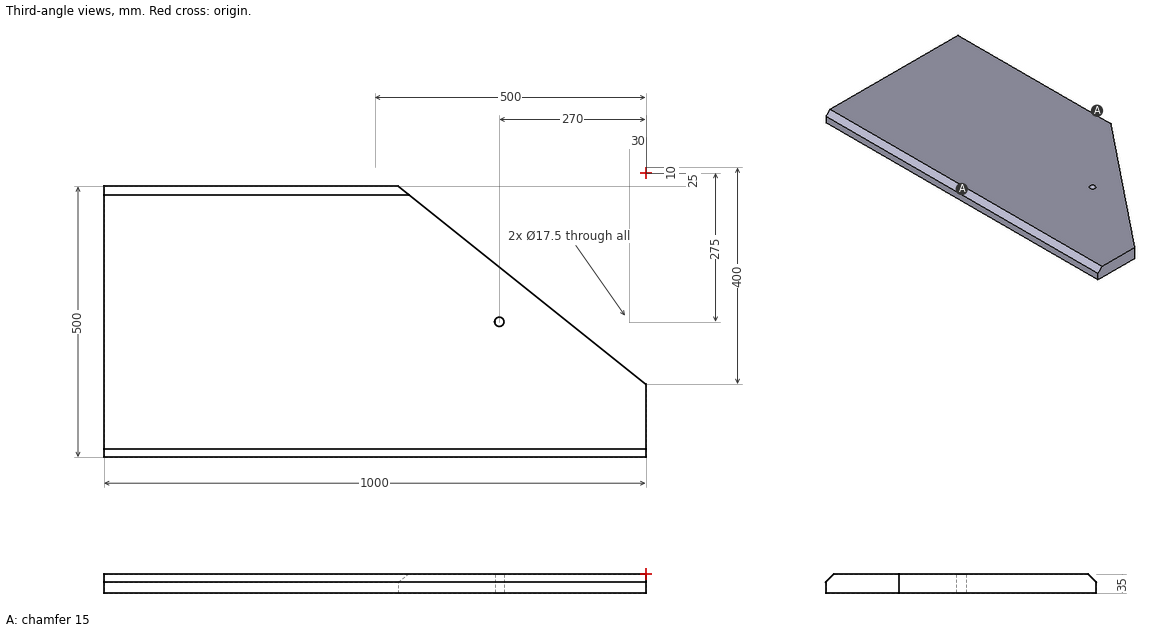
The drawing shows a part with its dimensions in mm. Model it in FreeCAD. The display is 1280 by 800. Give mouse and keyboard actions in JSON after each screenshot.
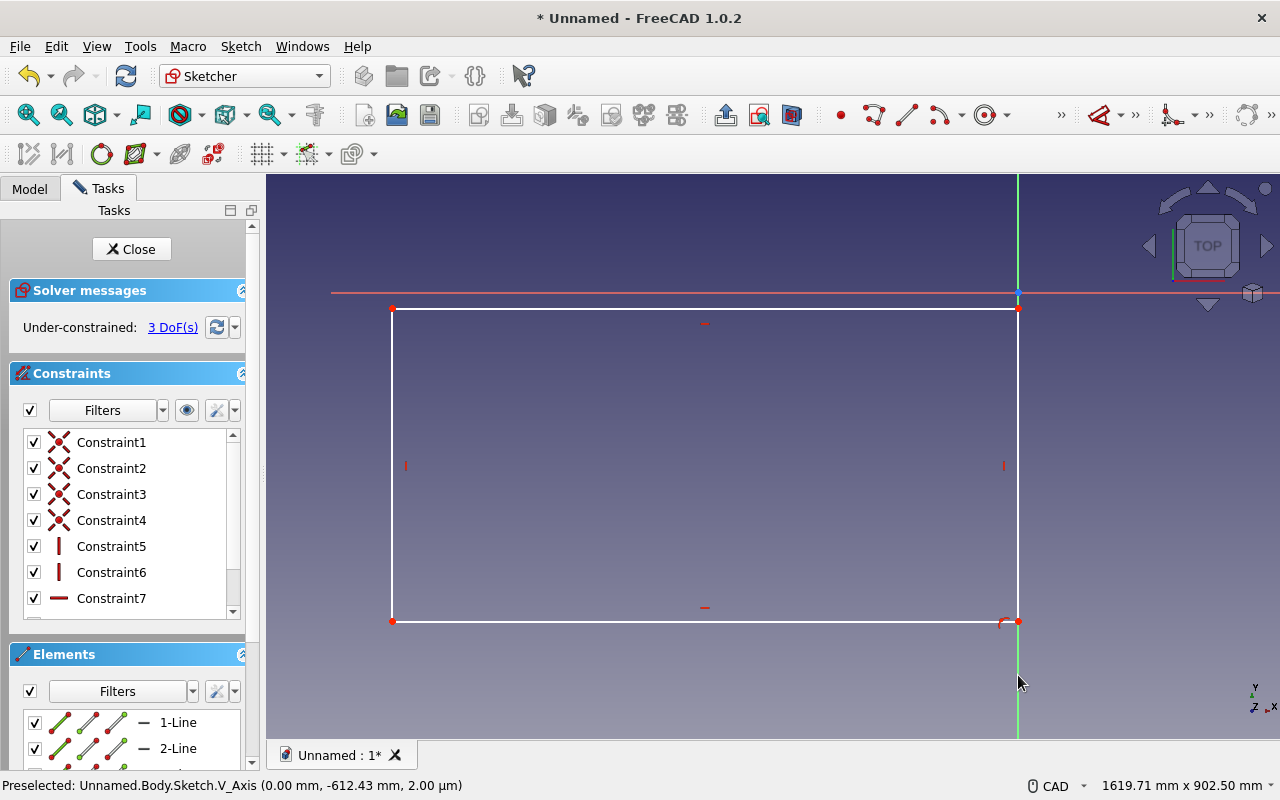
{"action": "left_click", "coordinate": [1098, 116]}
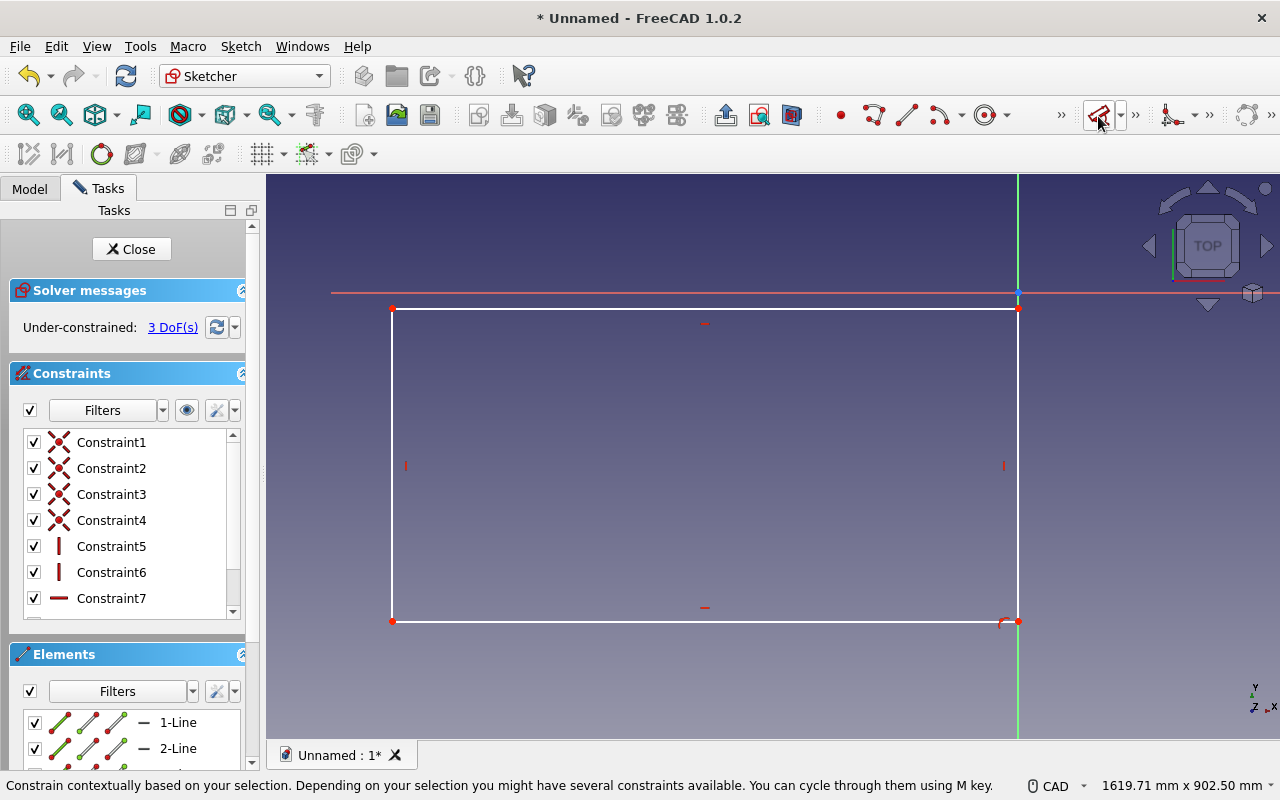
{"action": "left_click", "coordinate": [392, 403]}
{"action": "left_click", "coordinate": [358, 465]}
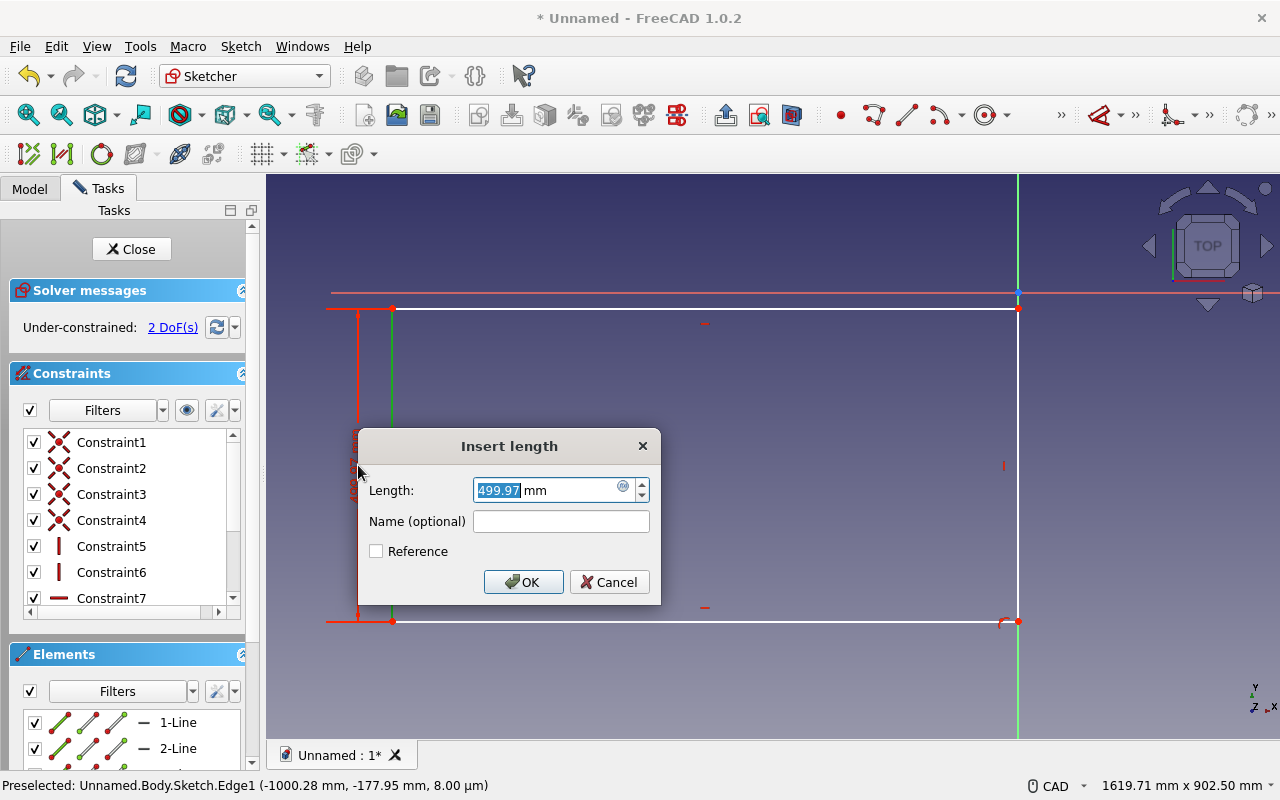
{"action": "type", "text": "500"}
{"action": "key", "text": "Return"}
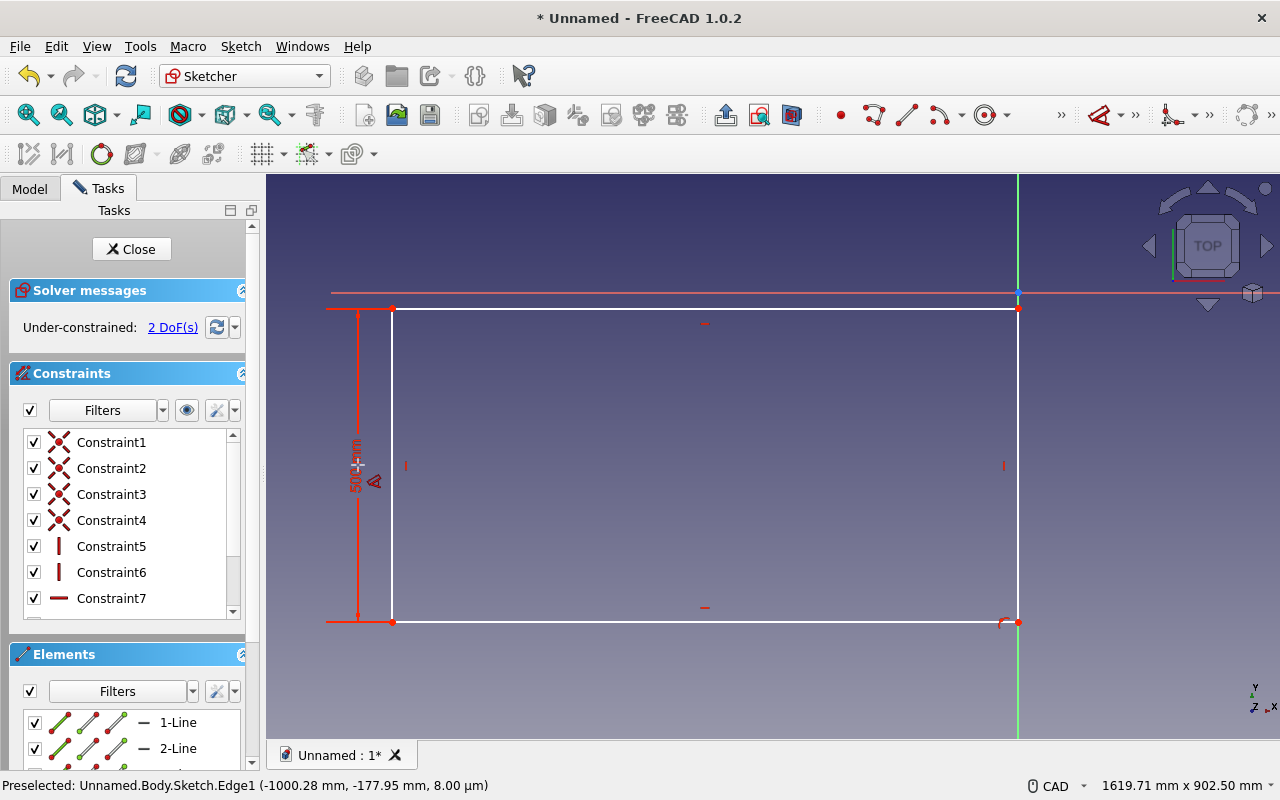
{"action": "scroll", "coordinate": [392, 309], "scroll_direction": "up", "scroll_amount": 5}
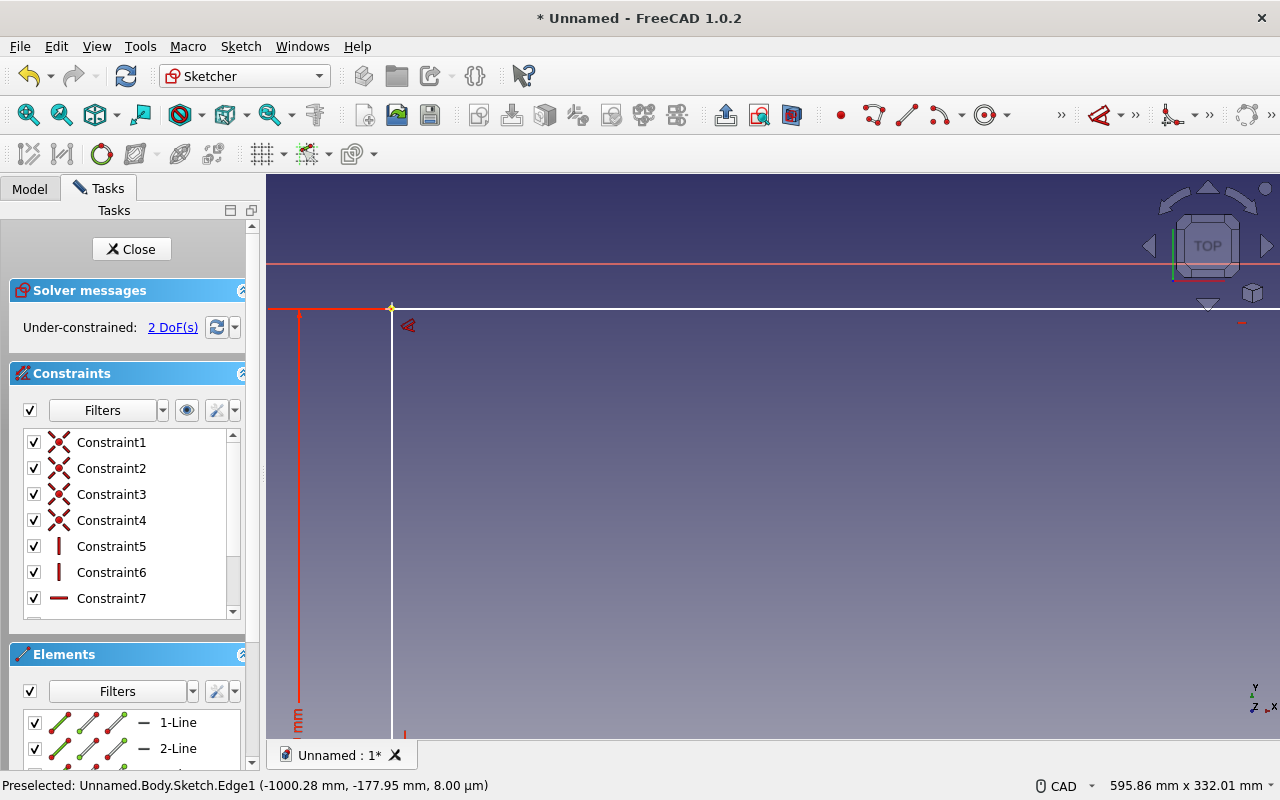
{"action": "left_click", "coordinate": [392, 309]}
{"action": "left_click", "coordinate": [358, 286]}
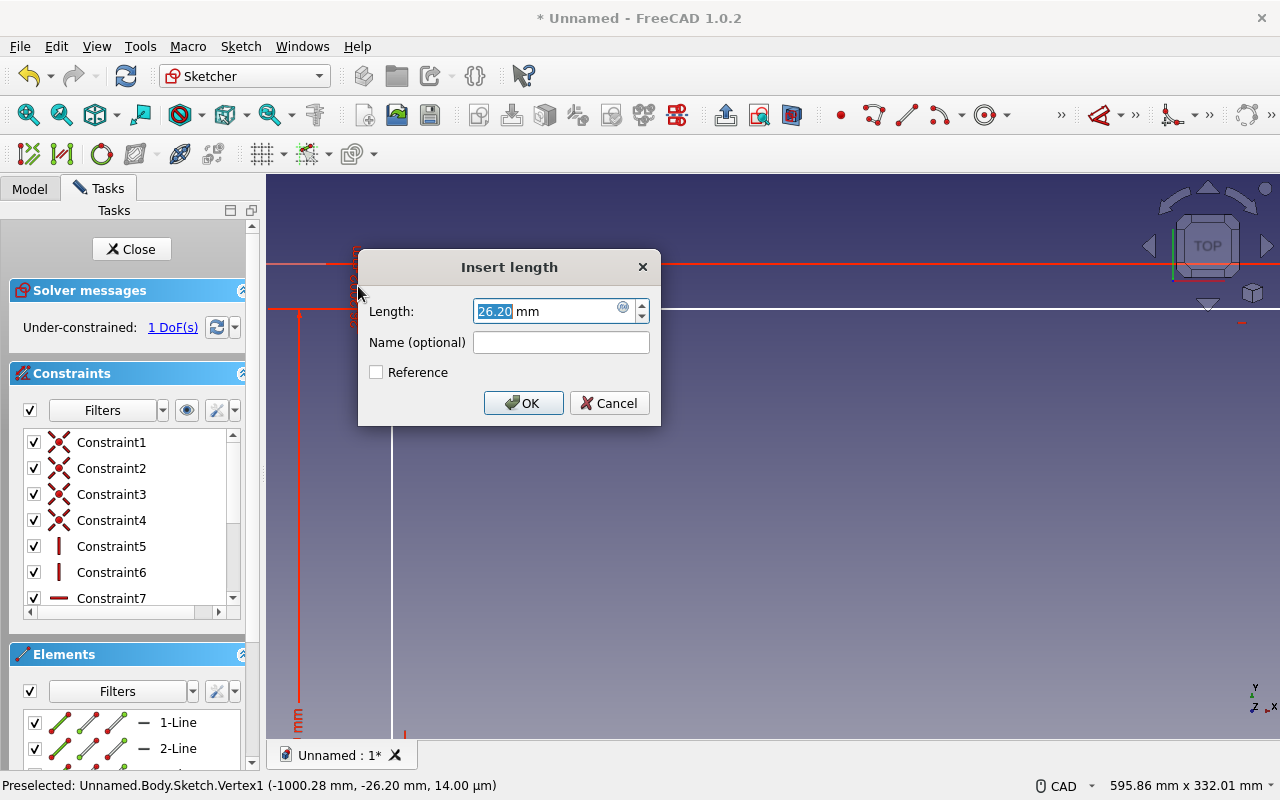
{"action": "type", "text": "25"}
{"action": "key", "text": "Return"}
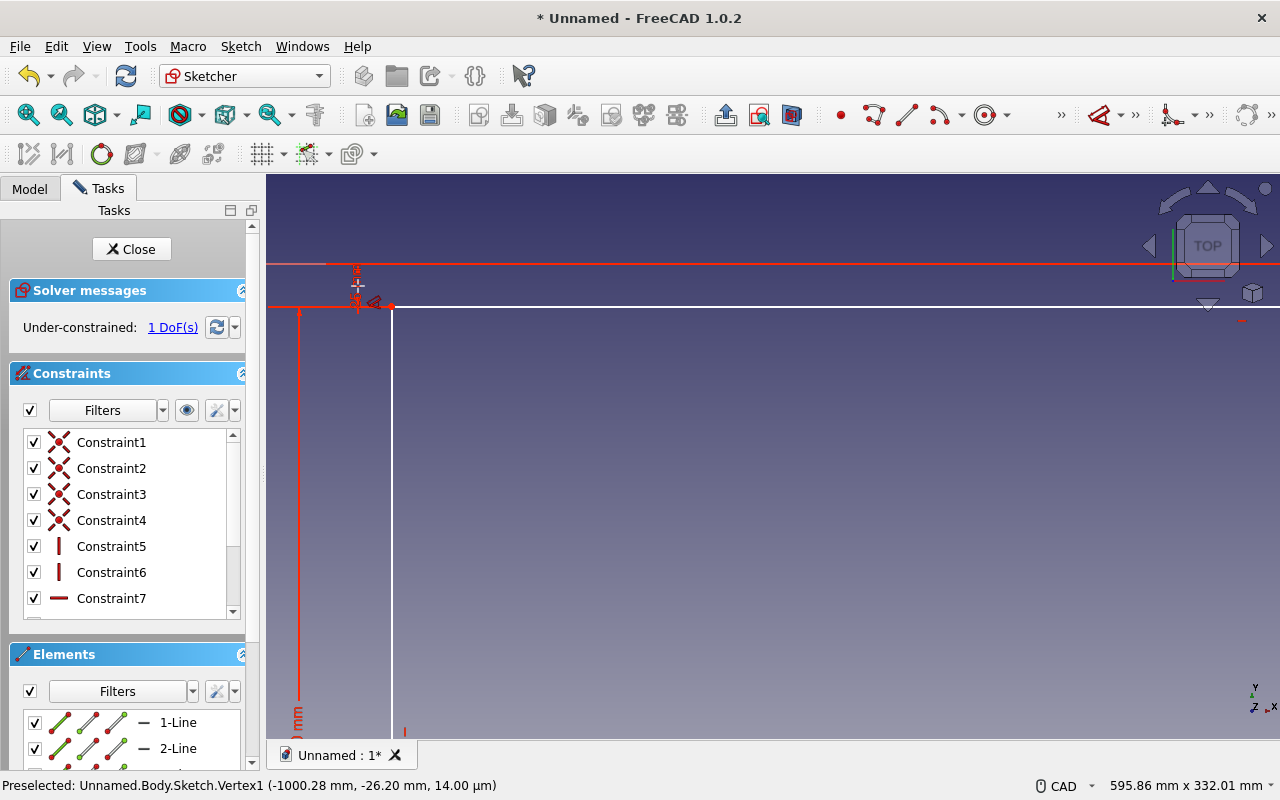
{"action": "scroll", "coordinate": [391, 309], "scroll_direction": "down", "scroll_amount": 5}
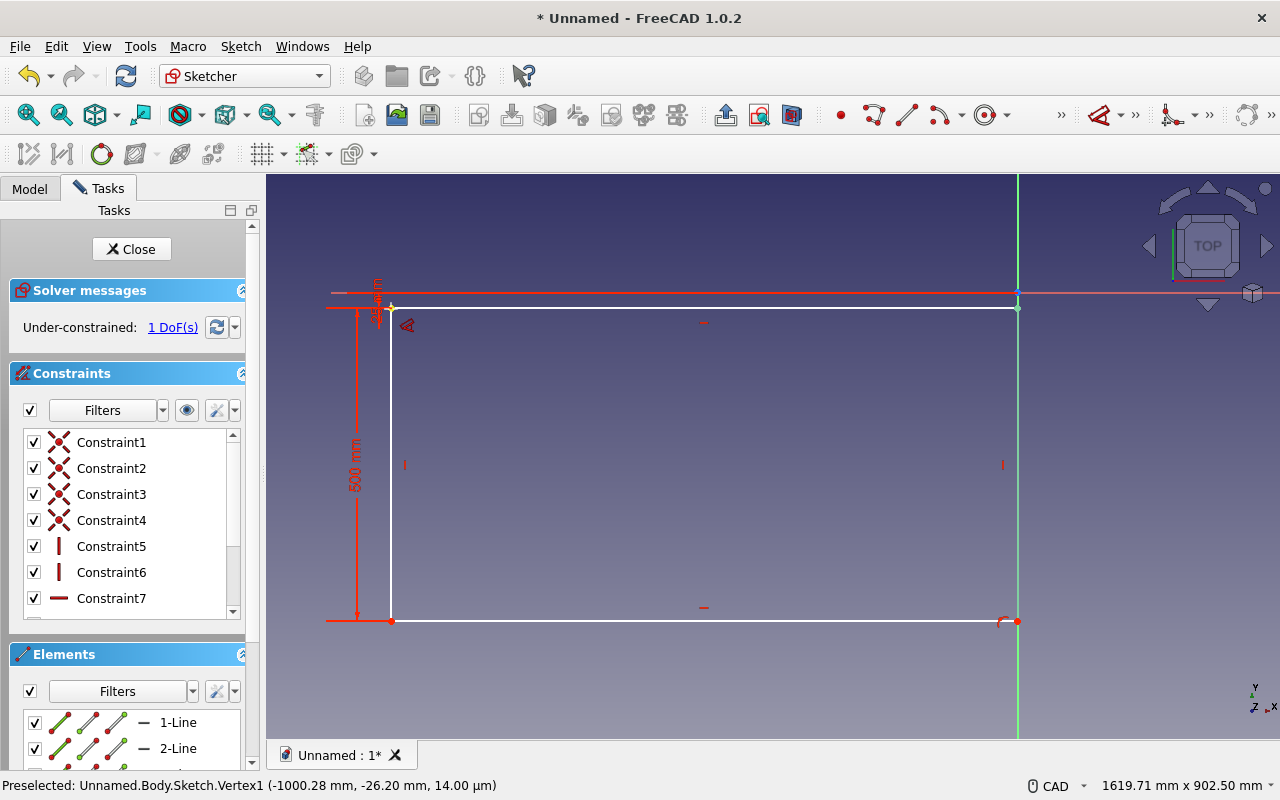
{"action": "left_click", "coordinate": [579, 621]}
{"action": "left_click", "coordinate": [704, 655]}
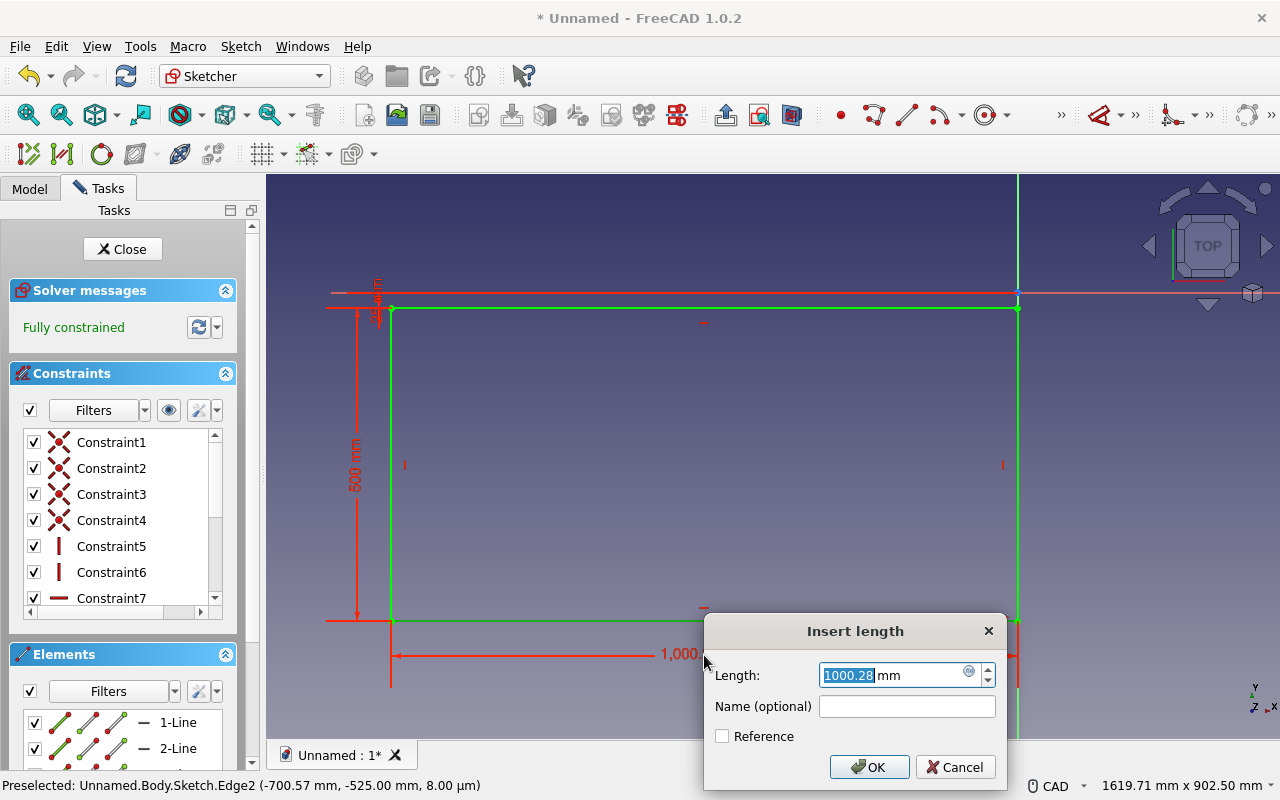
{"action": "type", "text": "1000"}
{"action": "key", "text": "Return"}
{"action": "key", "text": "Escape"}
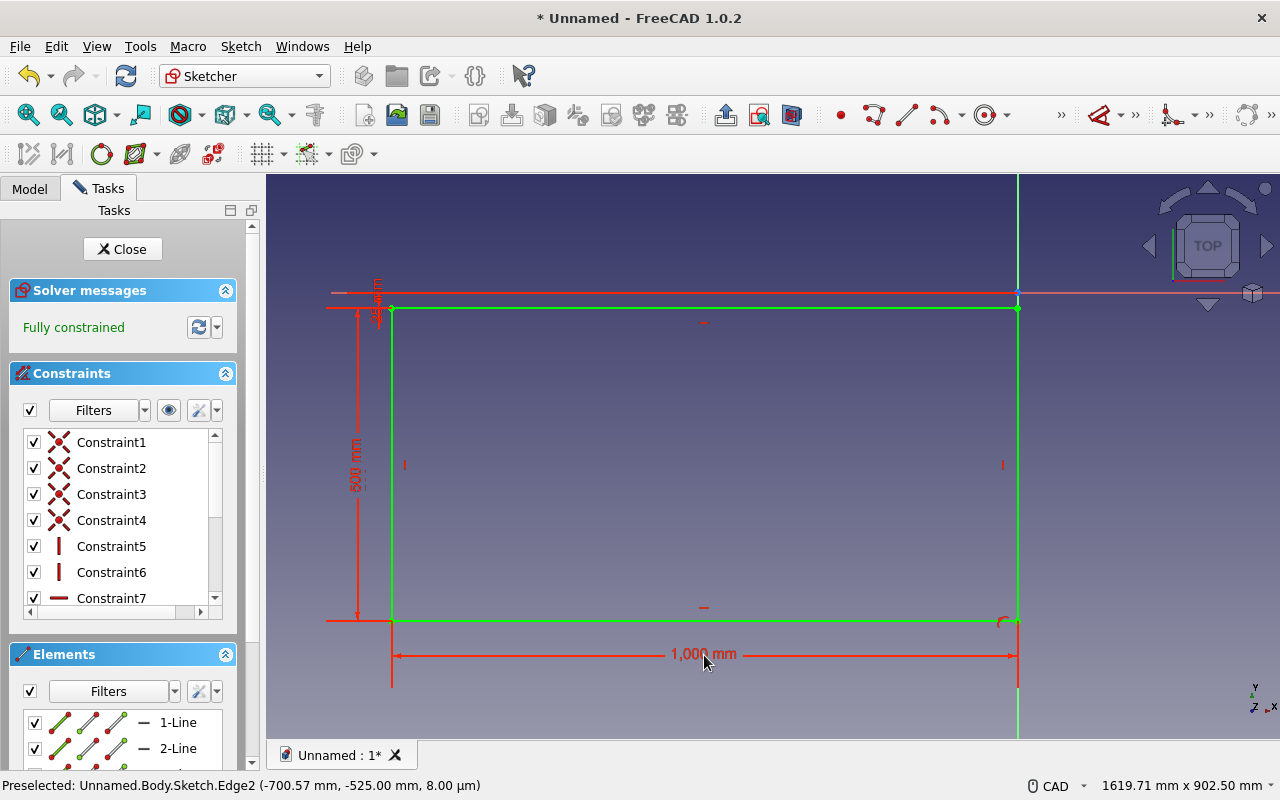
{"action": "left_click", "coordinate": [123, 249]}